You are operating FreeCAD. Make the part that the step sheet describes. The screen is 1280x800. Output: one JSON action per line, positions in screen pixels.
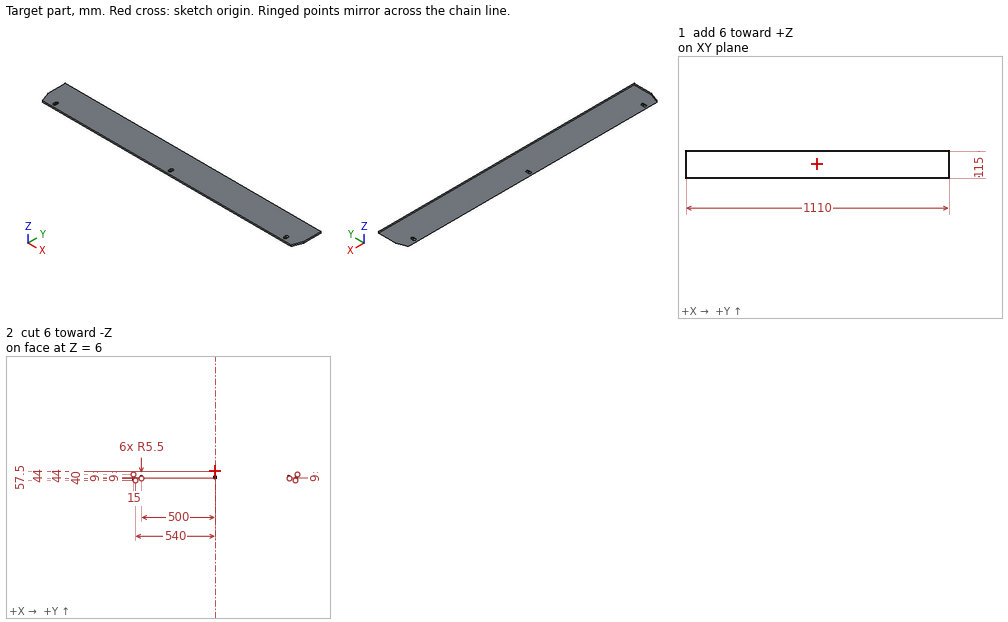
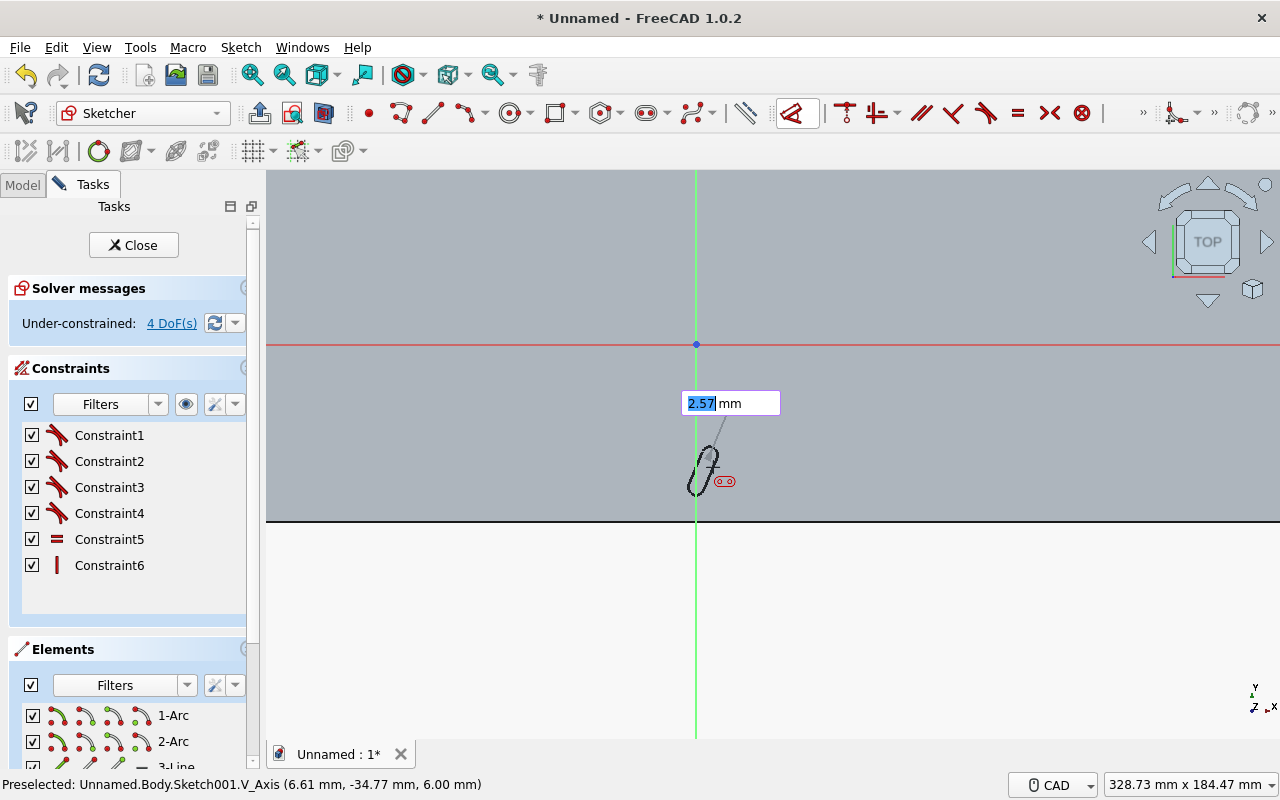
{"action": "left_click", "coordinate": [713, 467]}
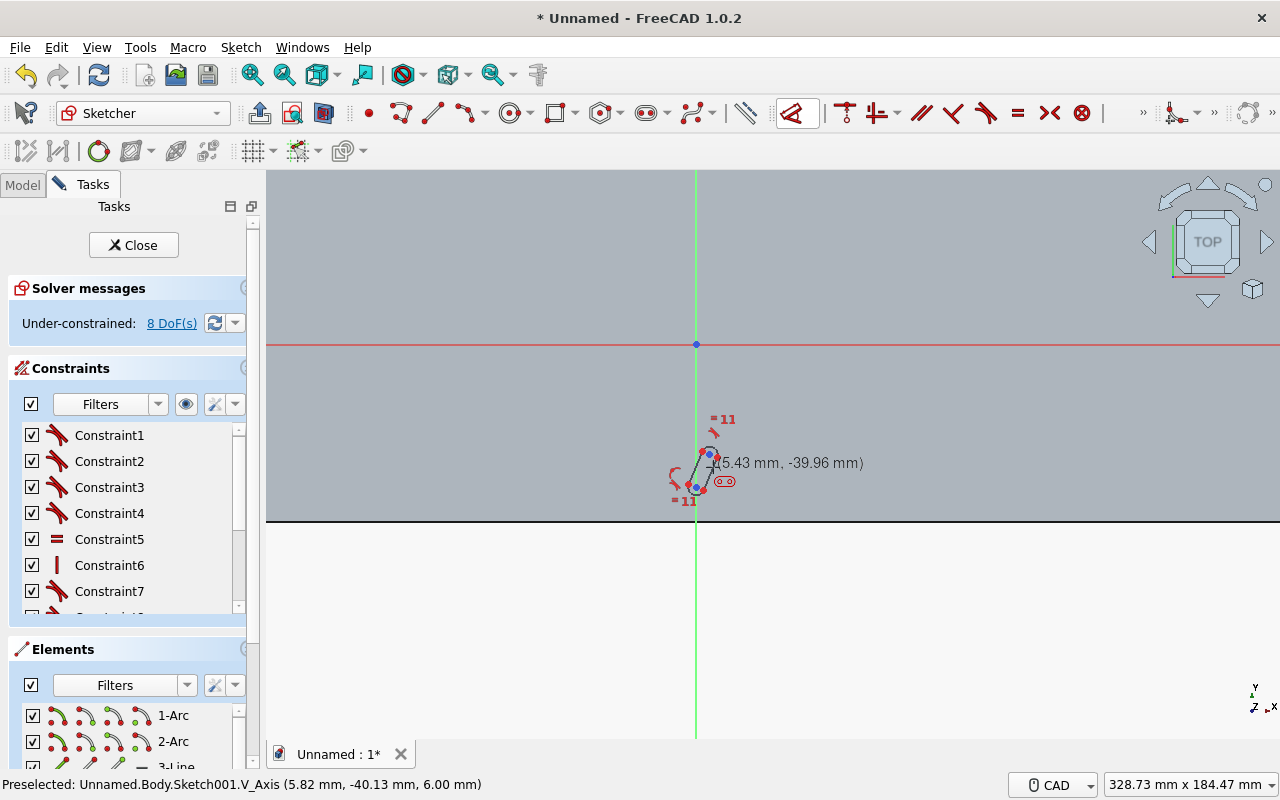
{"action": "scroll", "coordinate": [706, 459], "scroll_direction": "down", "scroll_amount": 9}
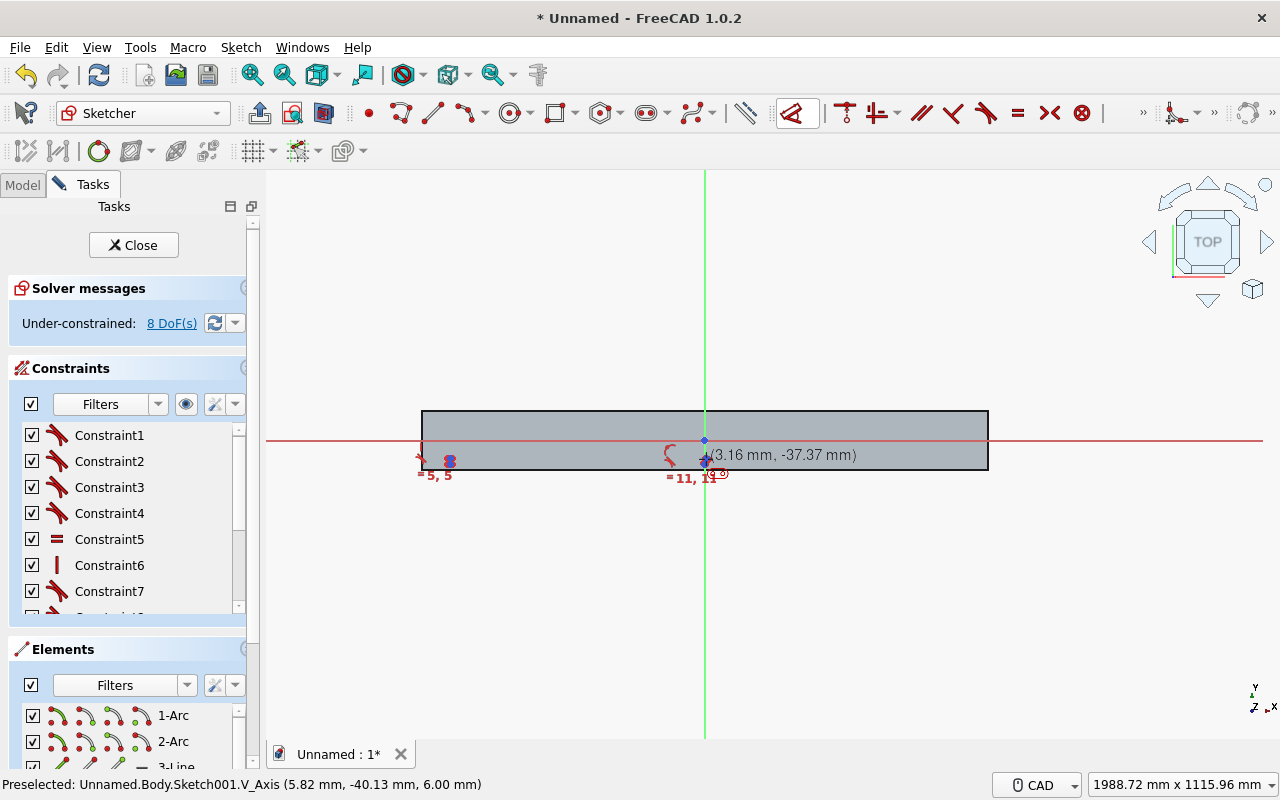
{"action": "scroll", "coordinate": [960, 463], "scroll_direction": "up", "scroll_amount": 11}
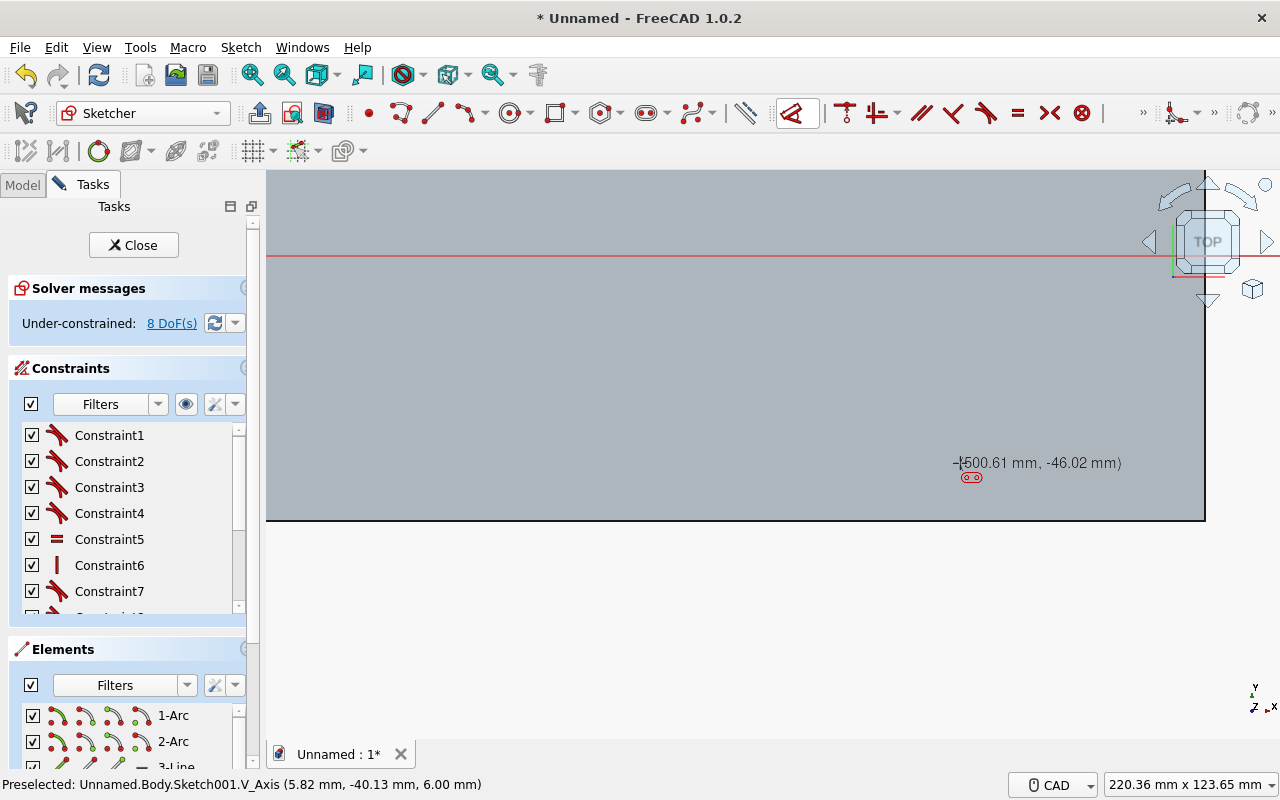
{"action": "scroll", "coordinate": [960, 463], "scroll_direction": "down", "scroll_amount": 11}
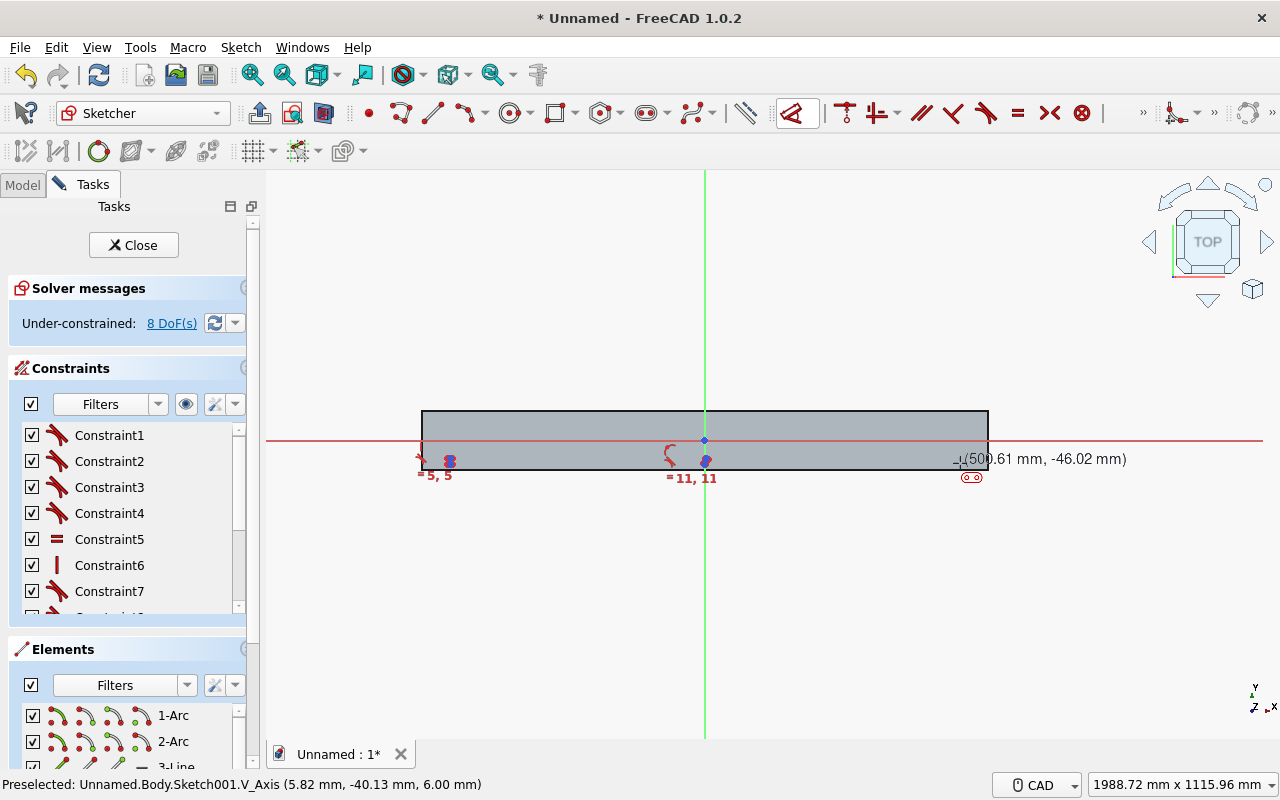
{"action": "left_click", "coordinate": [960, 463]}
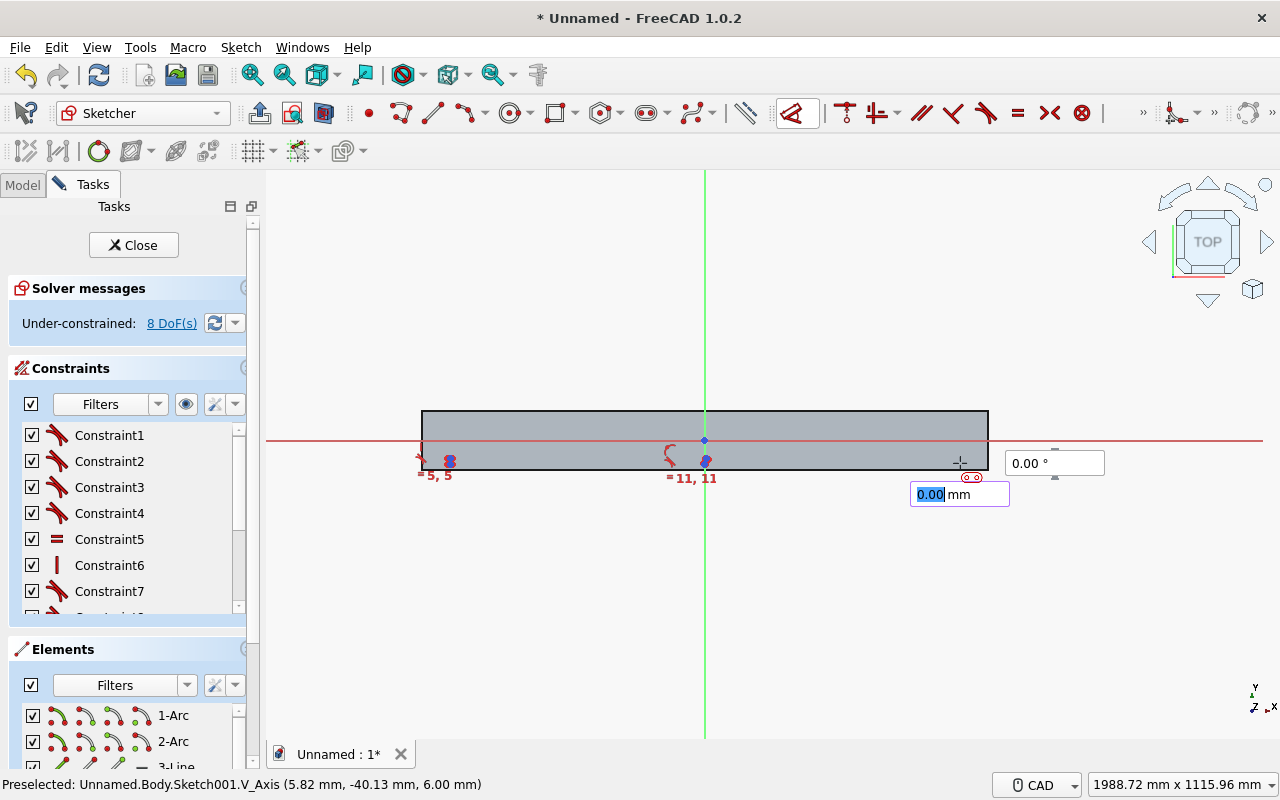
{"action": "scroll", "coordinate": [960, 458], "scroll_direction": "up", "scroll_amount": 7}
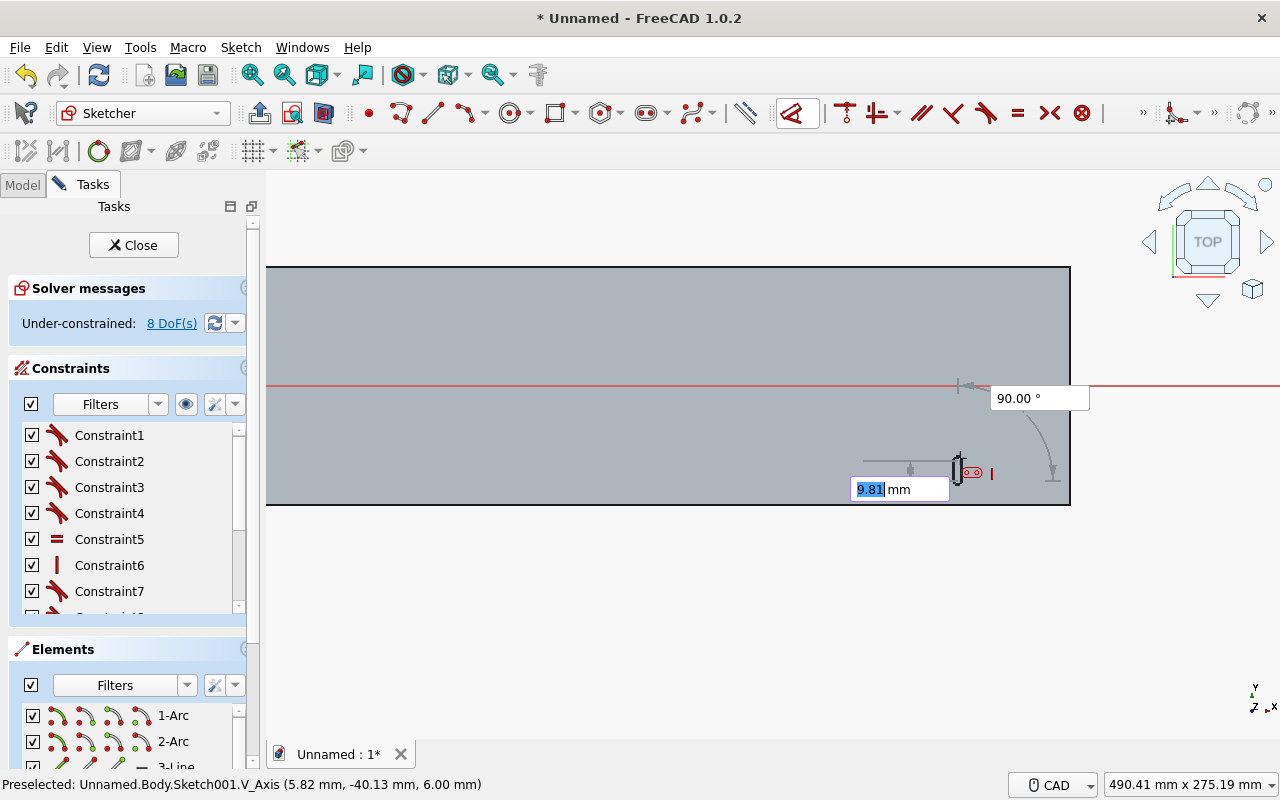
{"action": "left_click", "coordinate": [958, 458]}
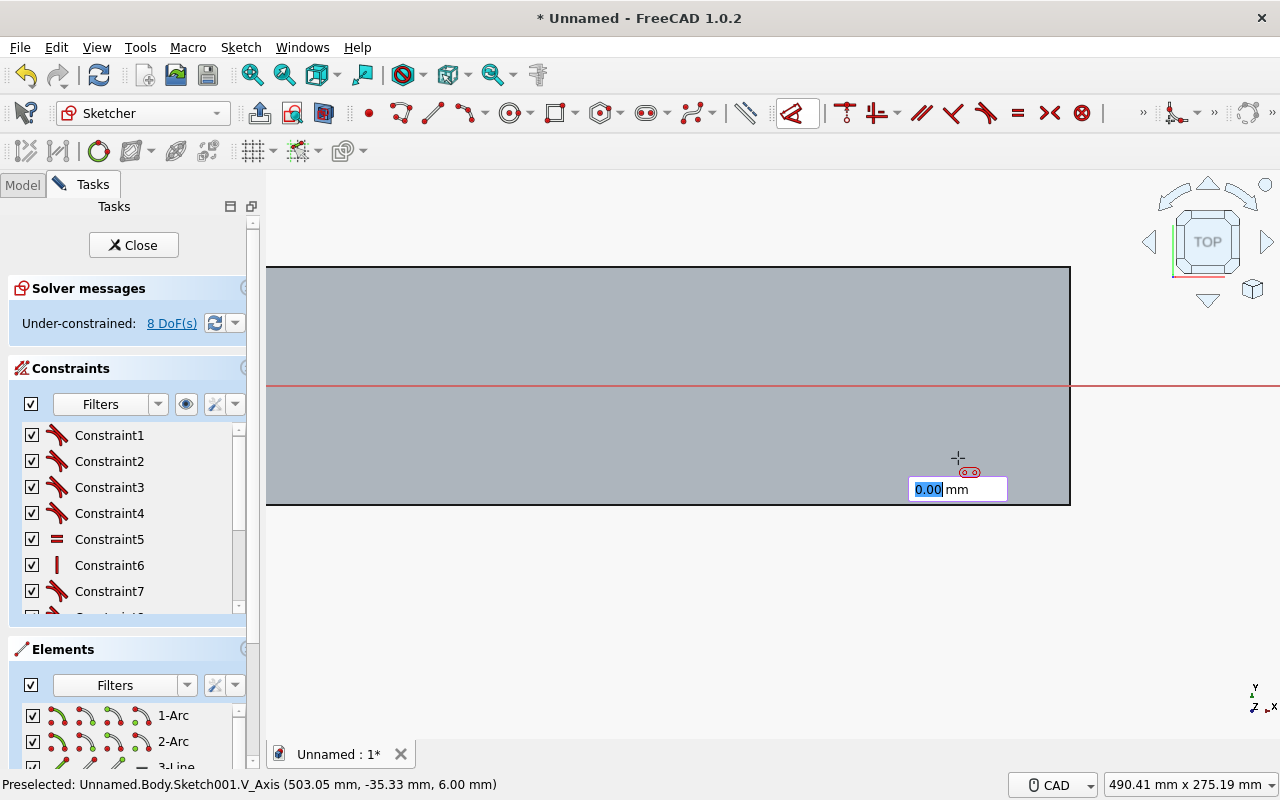
{"action": "scroll", "coordinate": [945, 467], "scroll_direction": "up", "scroll_amount": 2}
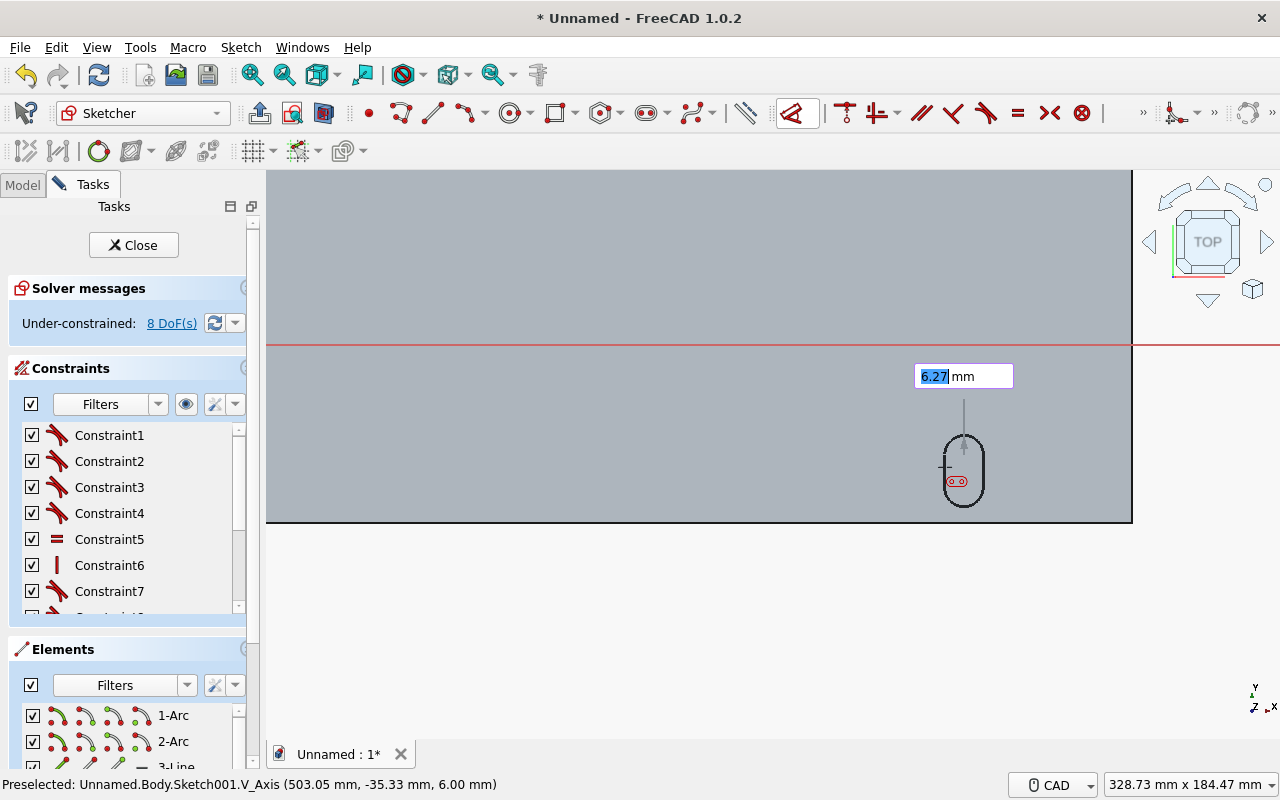
{"action": "left_click", "coordinate": [945, 467]}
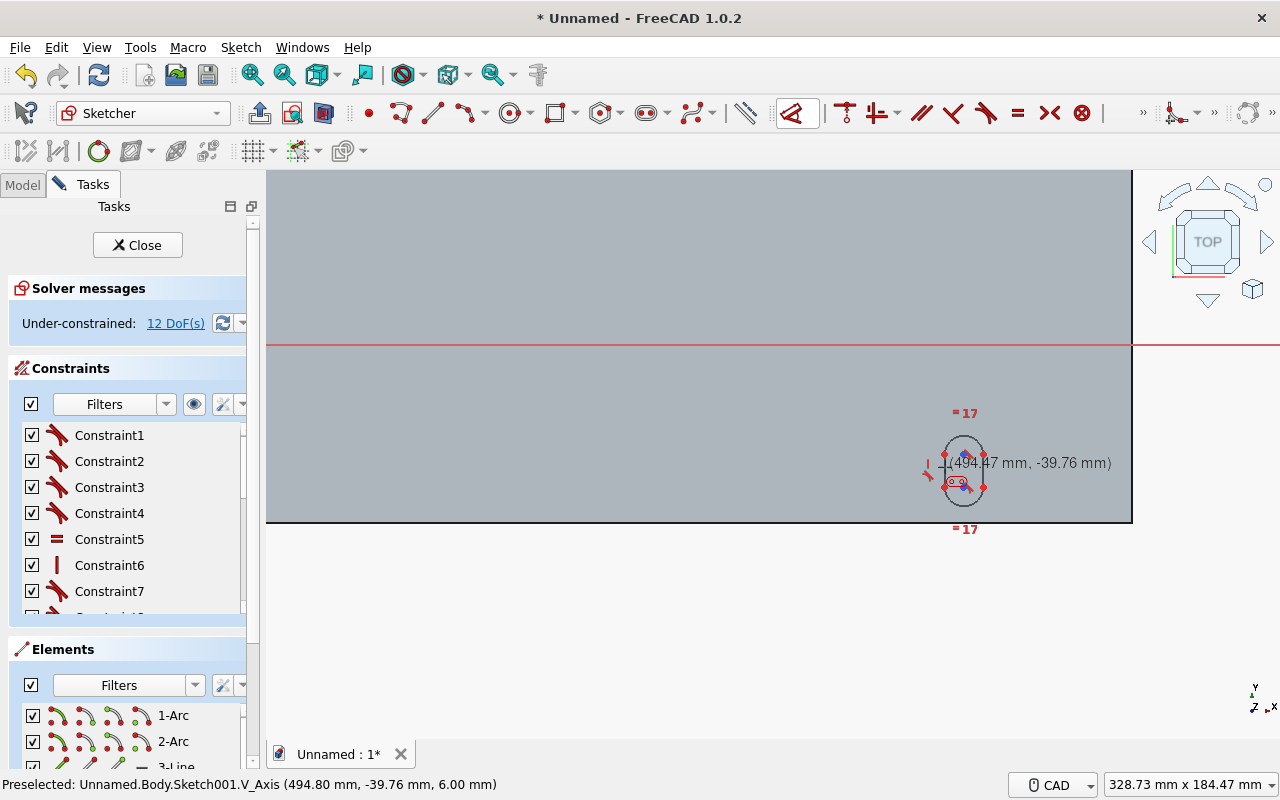
{"action": "left_click", "coordinate": [402, 114]}